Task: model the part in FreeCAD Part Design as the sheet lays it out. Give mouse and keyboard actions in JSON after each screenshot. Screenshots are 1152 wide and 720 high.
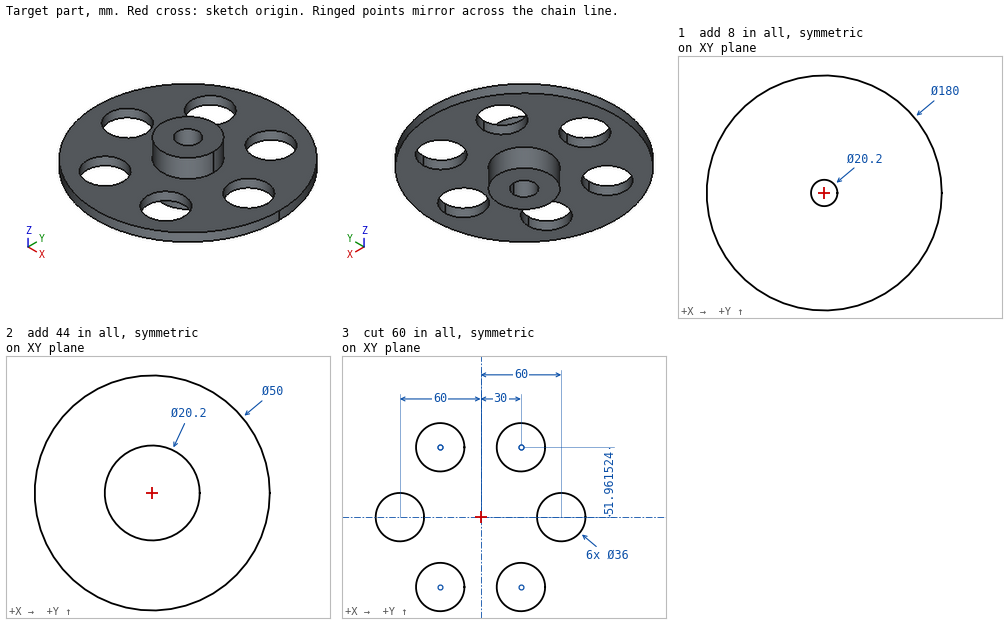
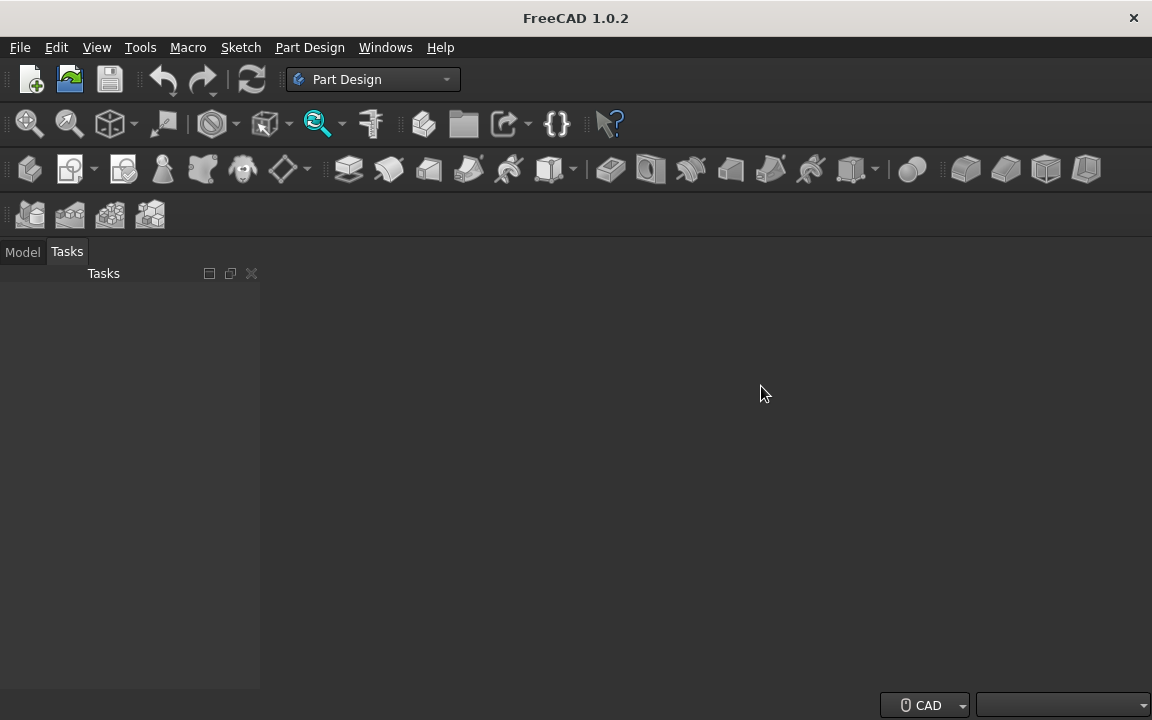
{"action": "key", "text": "ctrl+n"}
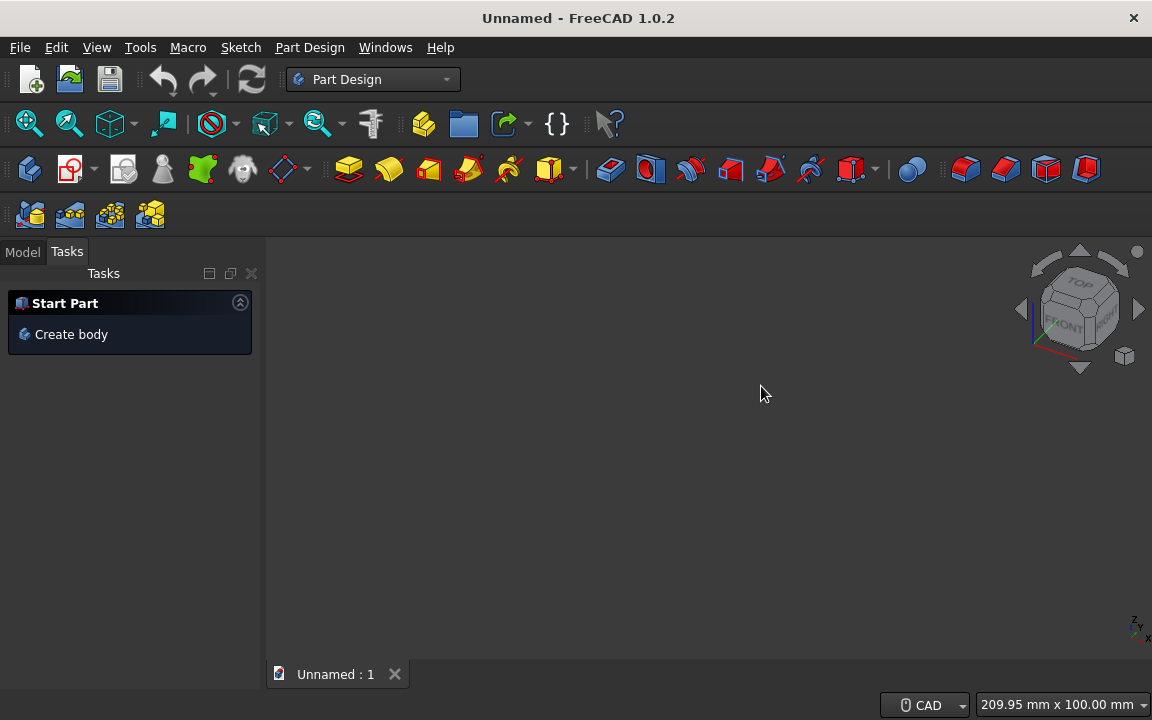
{"action": "left_click", "coordinate": [70, 170]}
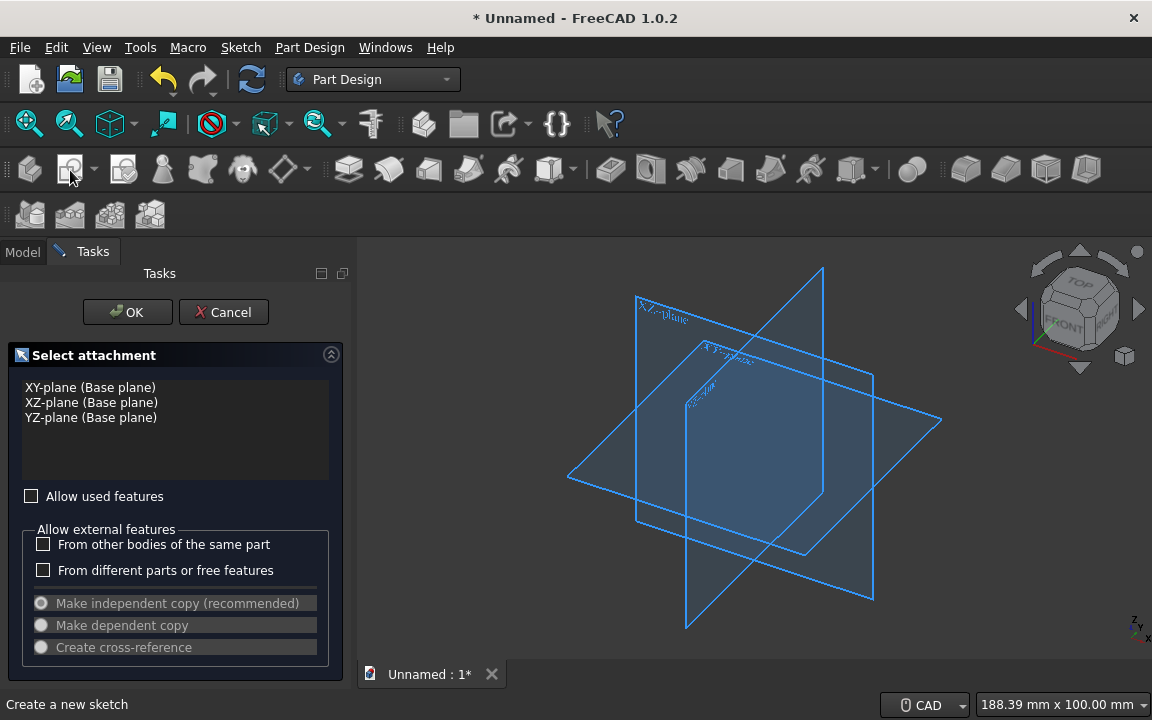
{"action": "left_click", "coordinate": [82, 388]}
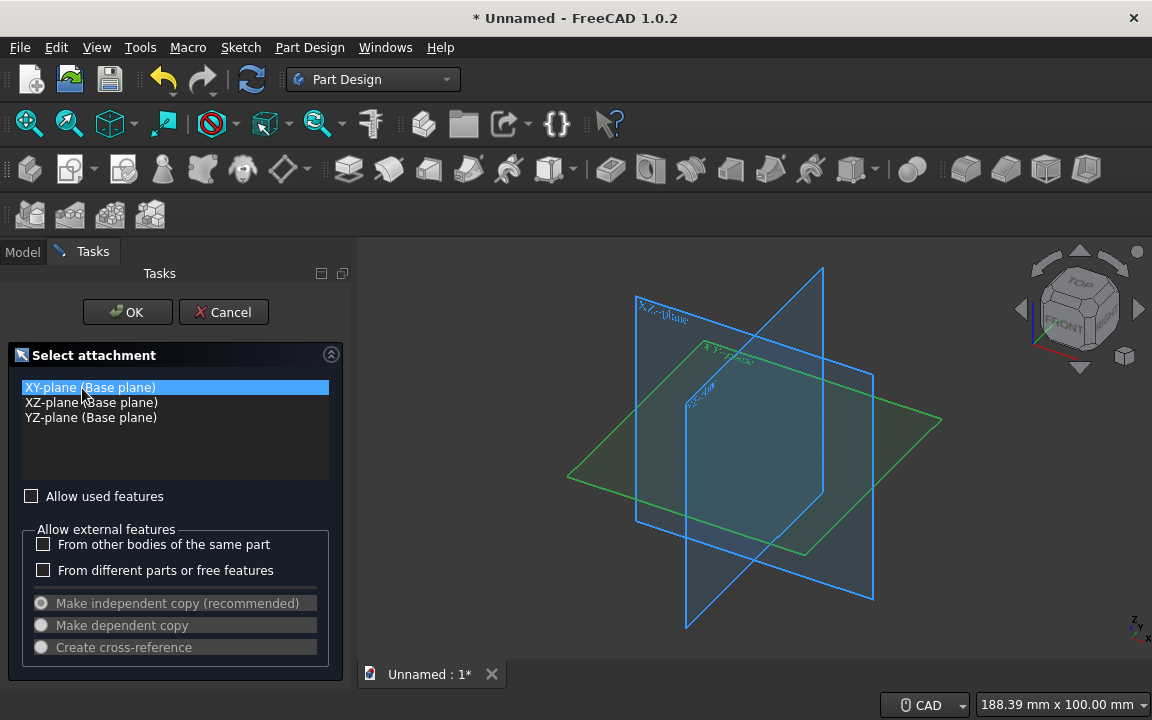
{"action": "left_click", "coordinate": [128, 312]}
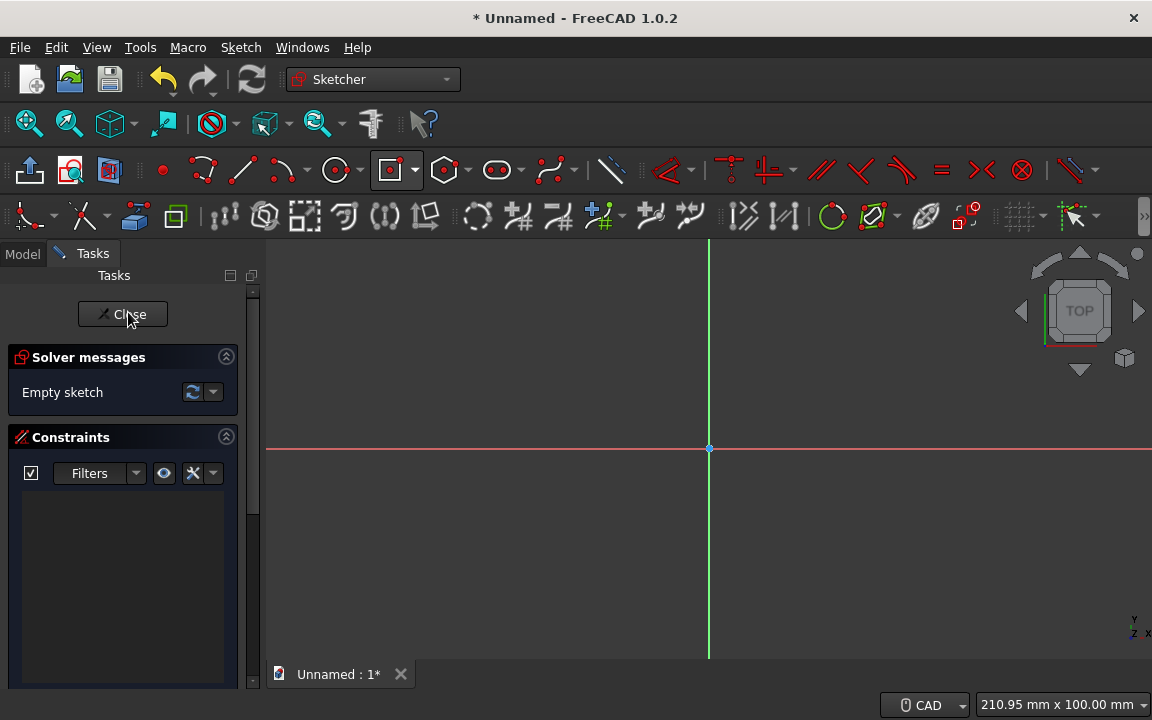
{"action": "scroll", "coordinate": [601, 449], "scroll_direction": "down", "scroll_amount": 5}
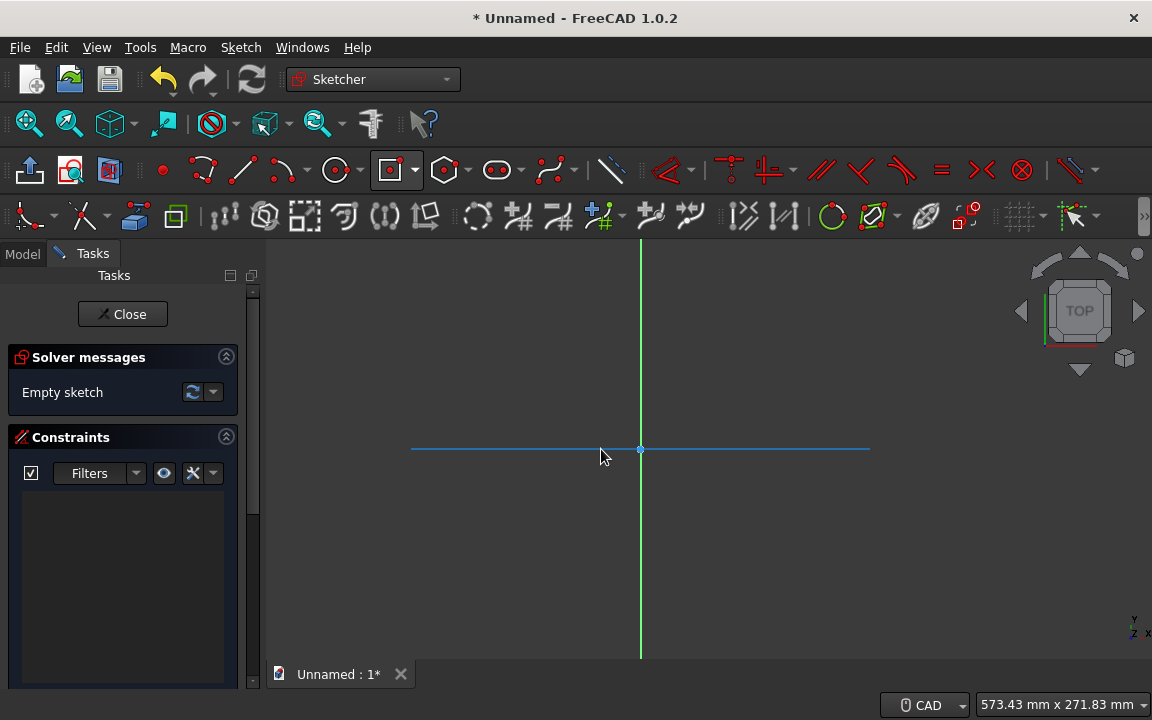
{"action": "key", "text": "g c"}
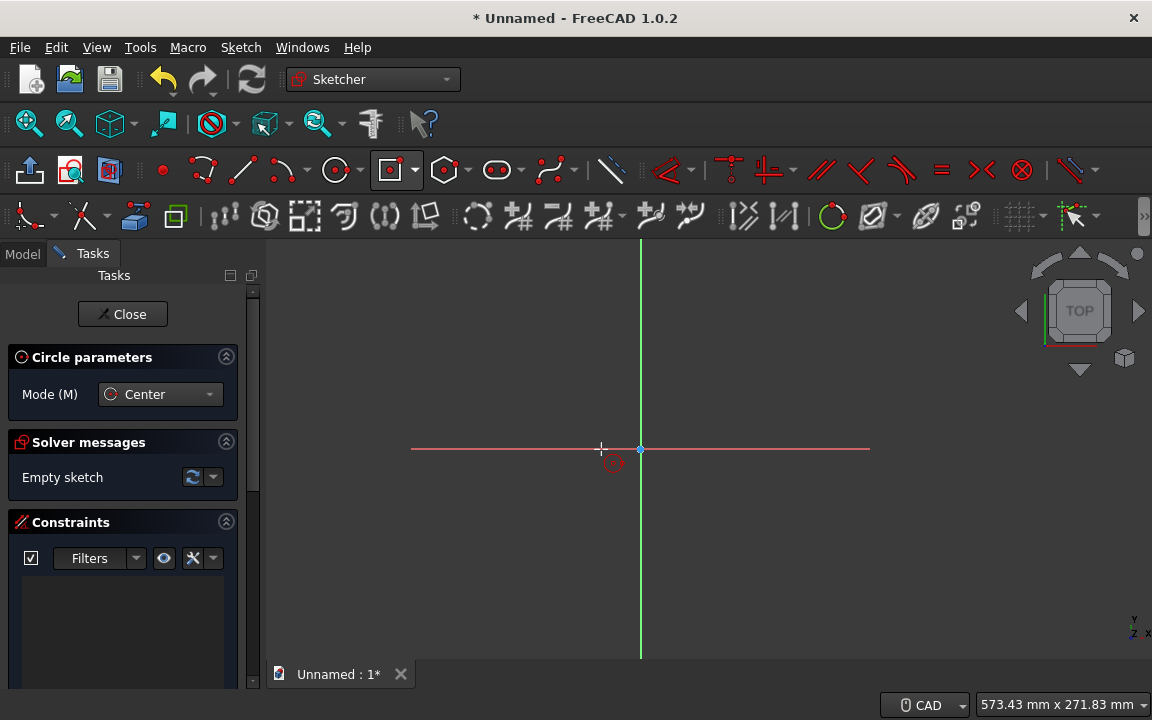
{"action": "left_click", "coordinate": [641, 449]}
{"action": "left_click", "coordinate": [739, 351]}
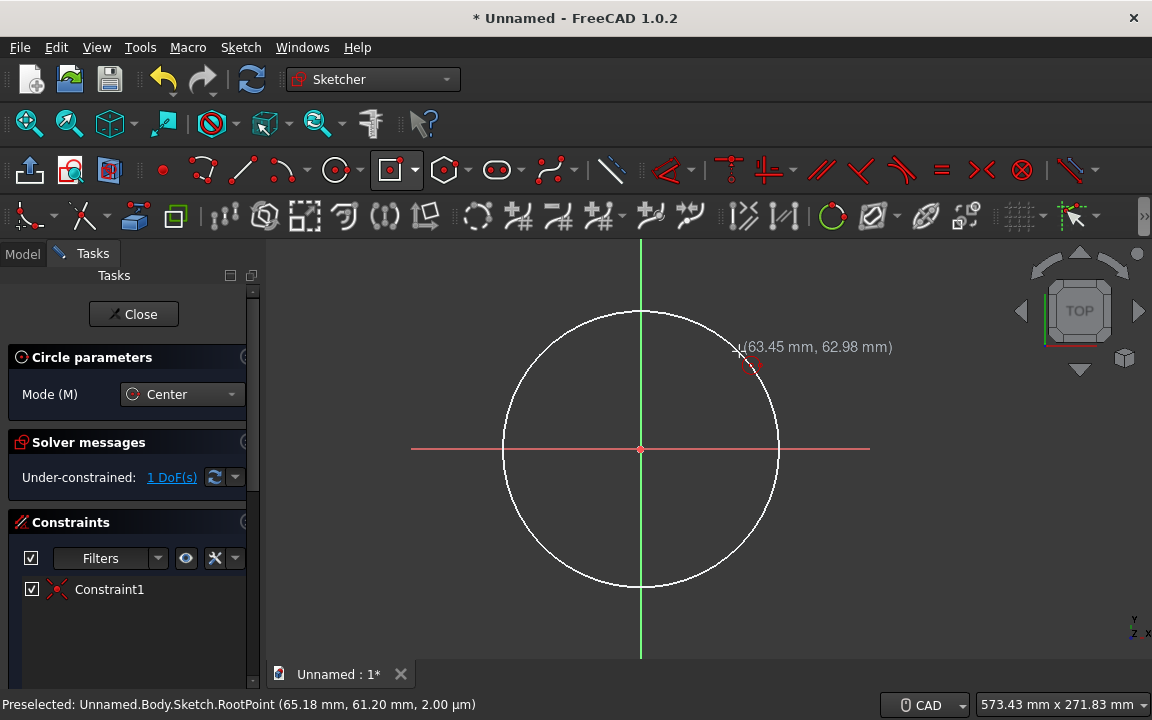
{"action": "scroll", "coordinate": [641, 449], "scroll_direction": "up", "scroll_amount": 2}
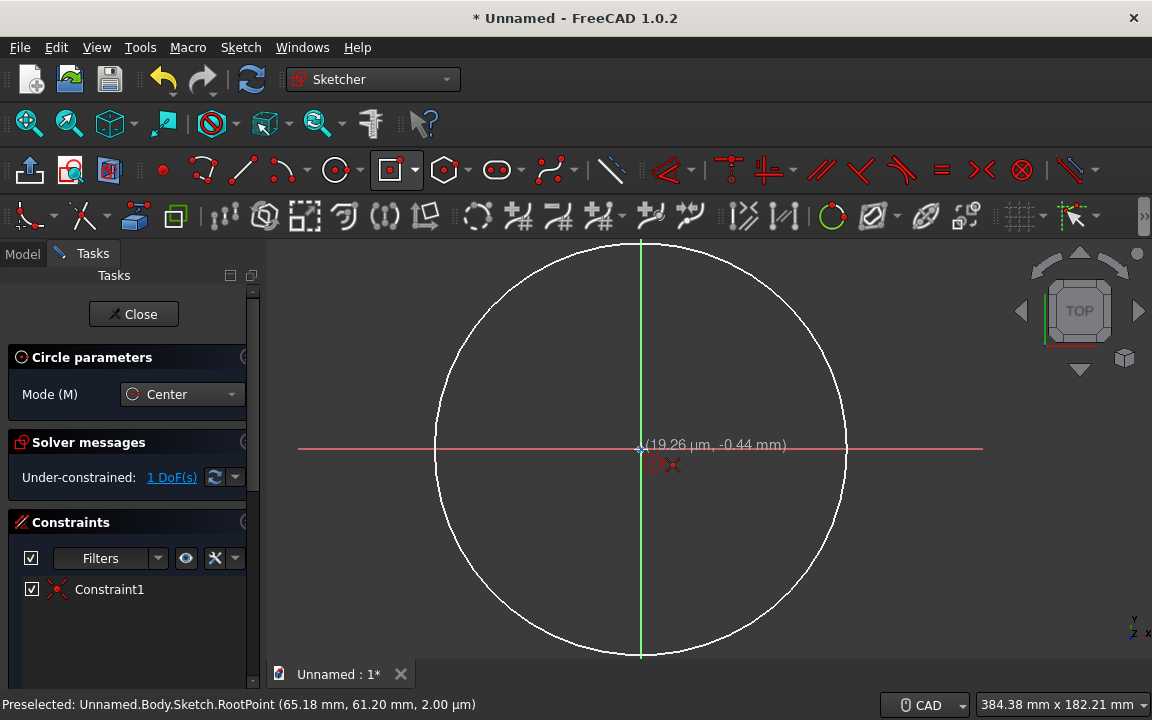
{"action": "left_click", "coordinate": [641, 449]}
{"action": "left_click", "coordinate": [657, 433]}
{"action": "key", "text": "Escape"}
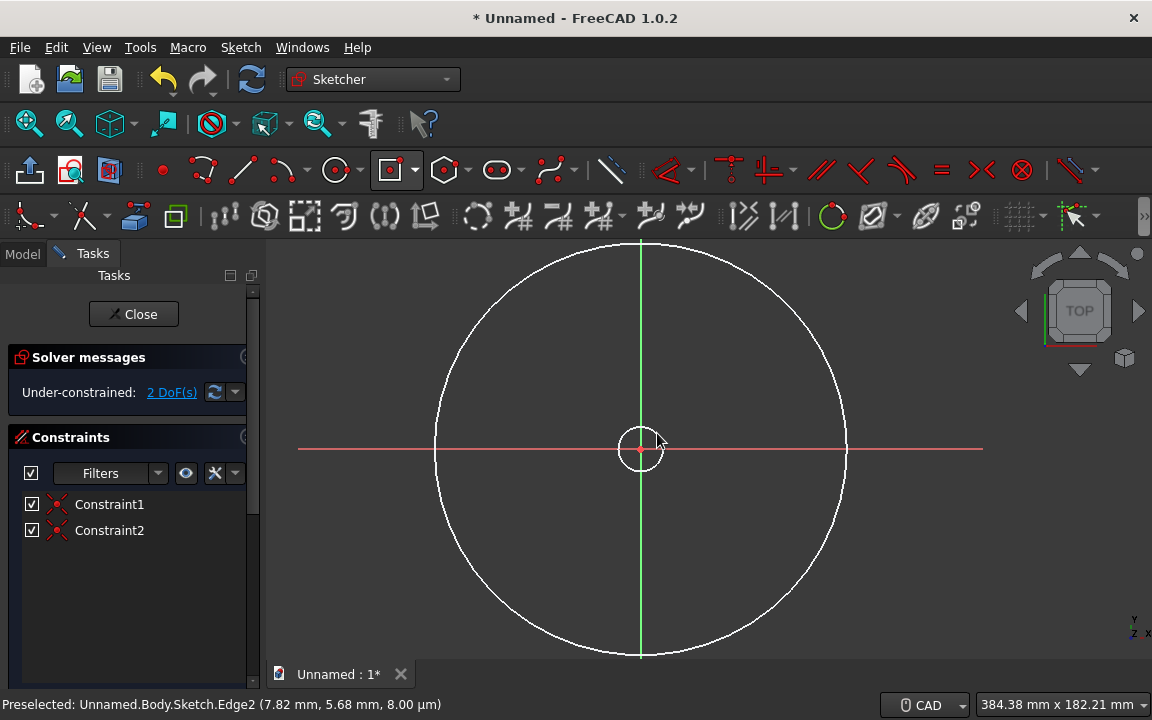
{"action": "left_click", "coordinate": [786, 303]}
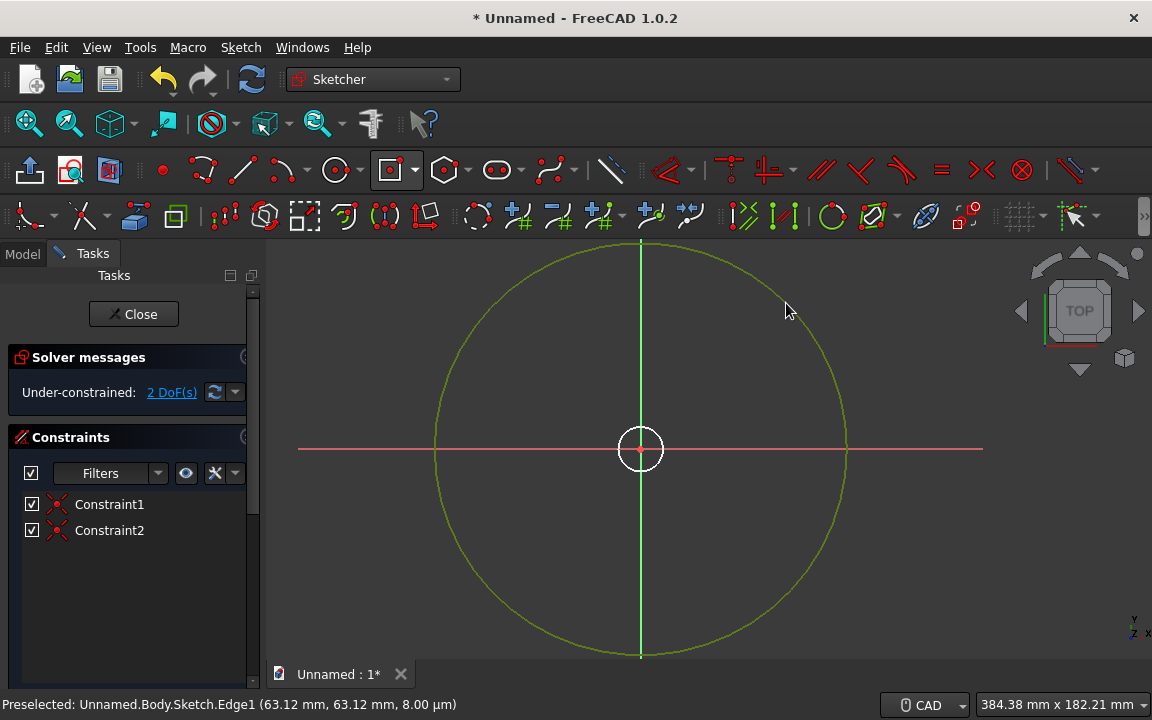
{"action": "key", "text": "k o"}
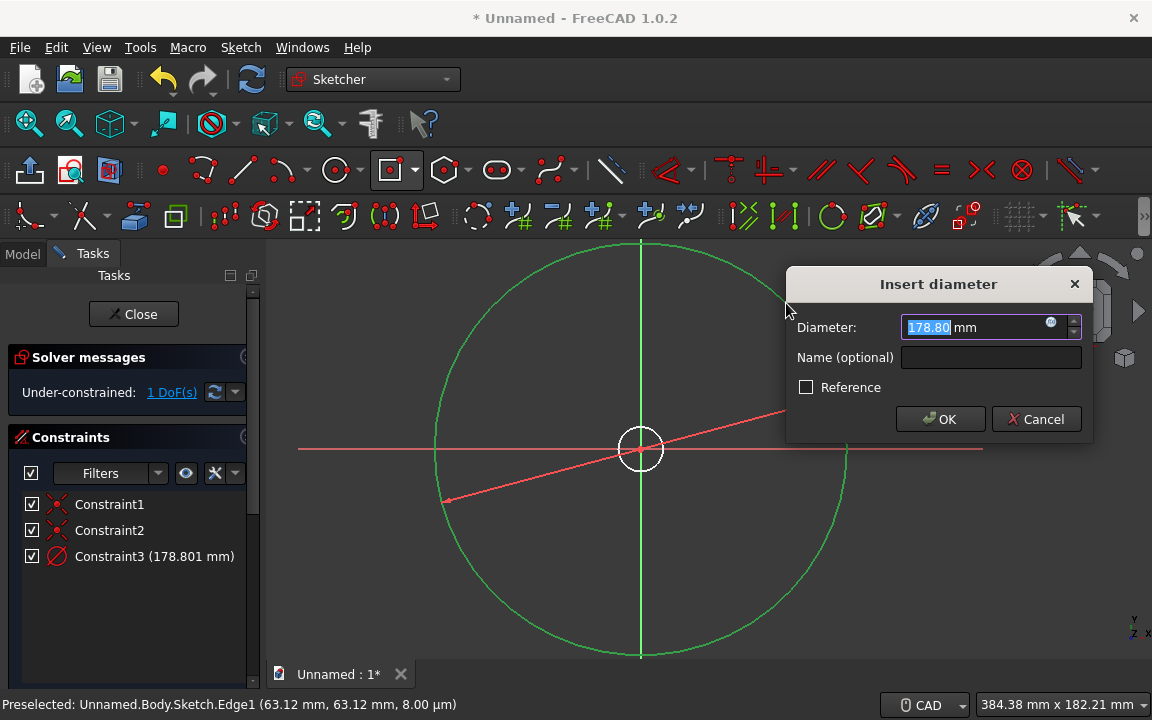
{"action": "type", "text": "180"}
{"action": "key", "text": "Return"}